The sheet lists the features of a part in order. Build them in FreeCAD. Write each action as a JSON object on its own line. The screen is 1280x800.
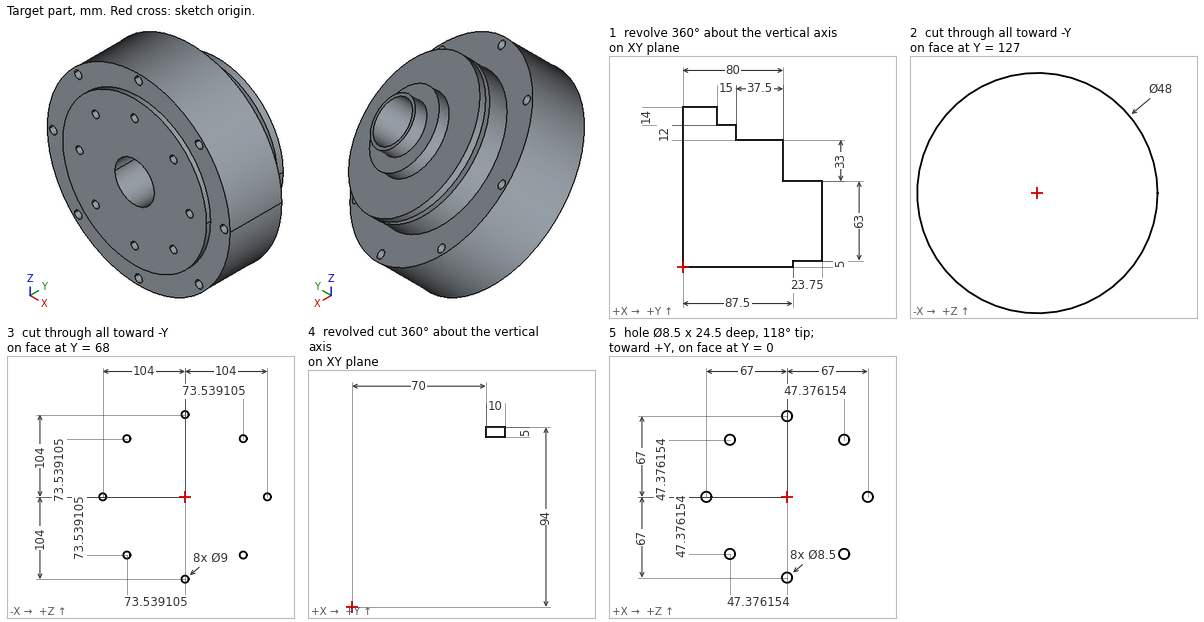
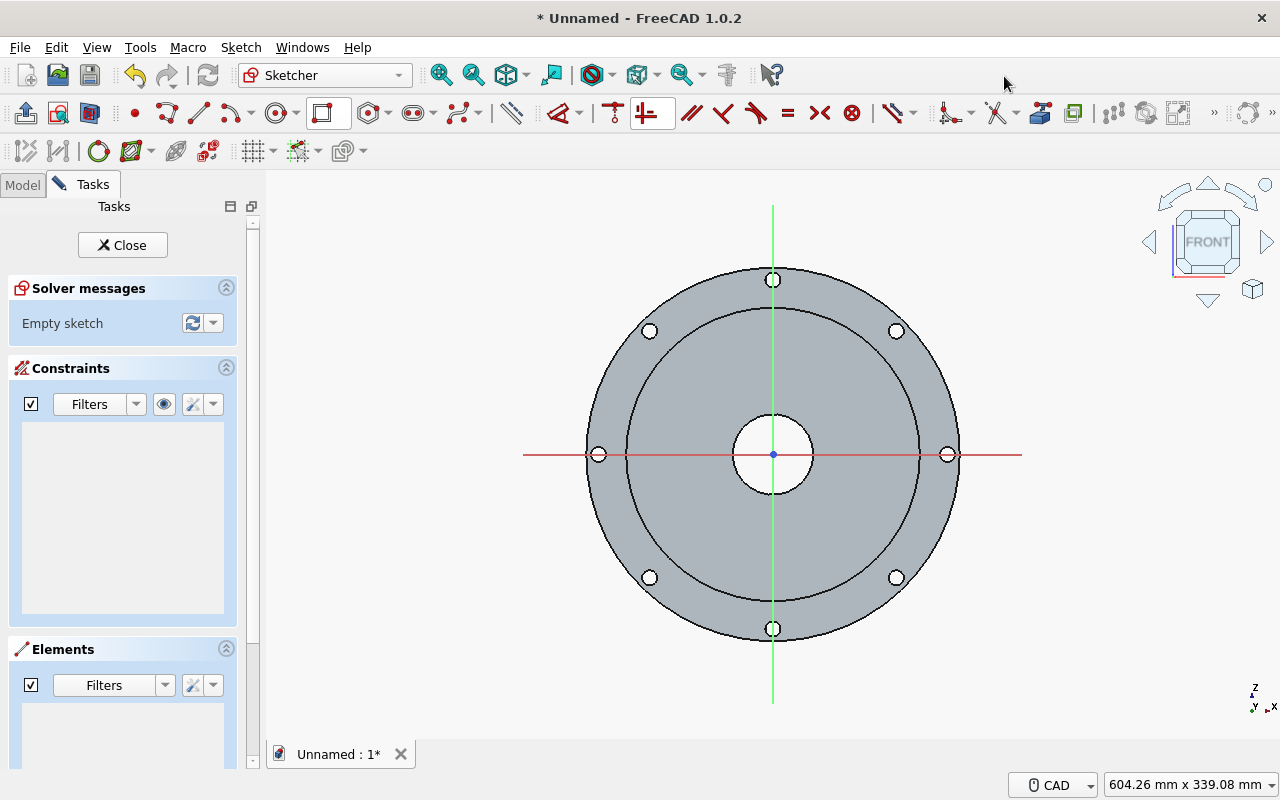
{"action": "scroll", "coordinate": [912, 455], "scroll_direction": "up", "scroll_amount": 2}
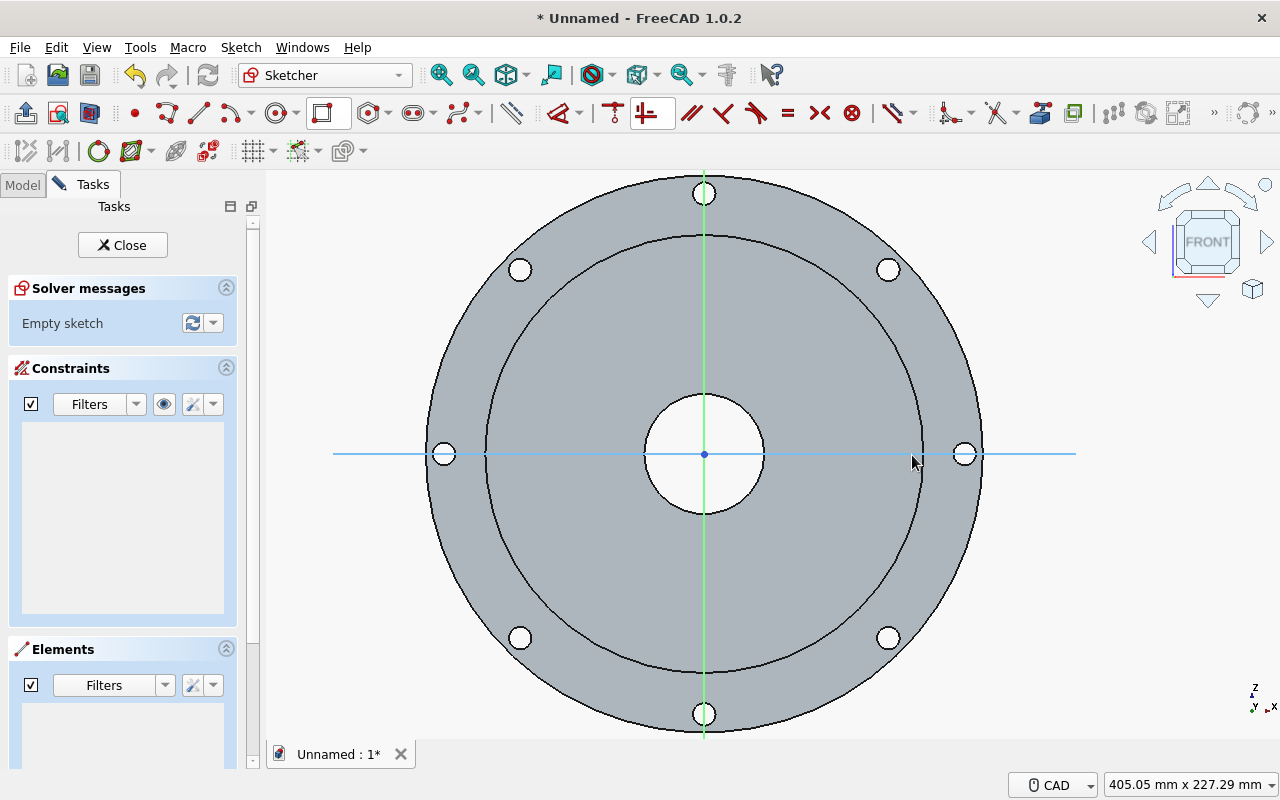
{"action": "left_click", "coordinate": [276, 114]}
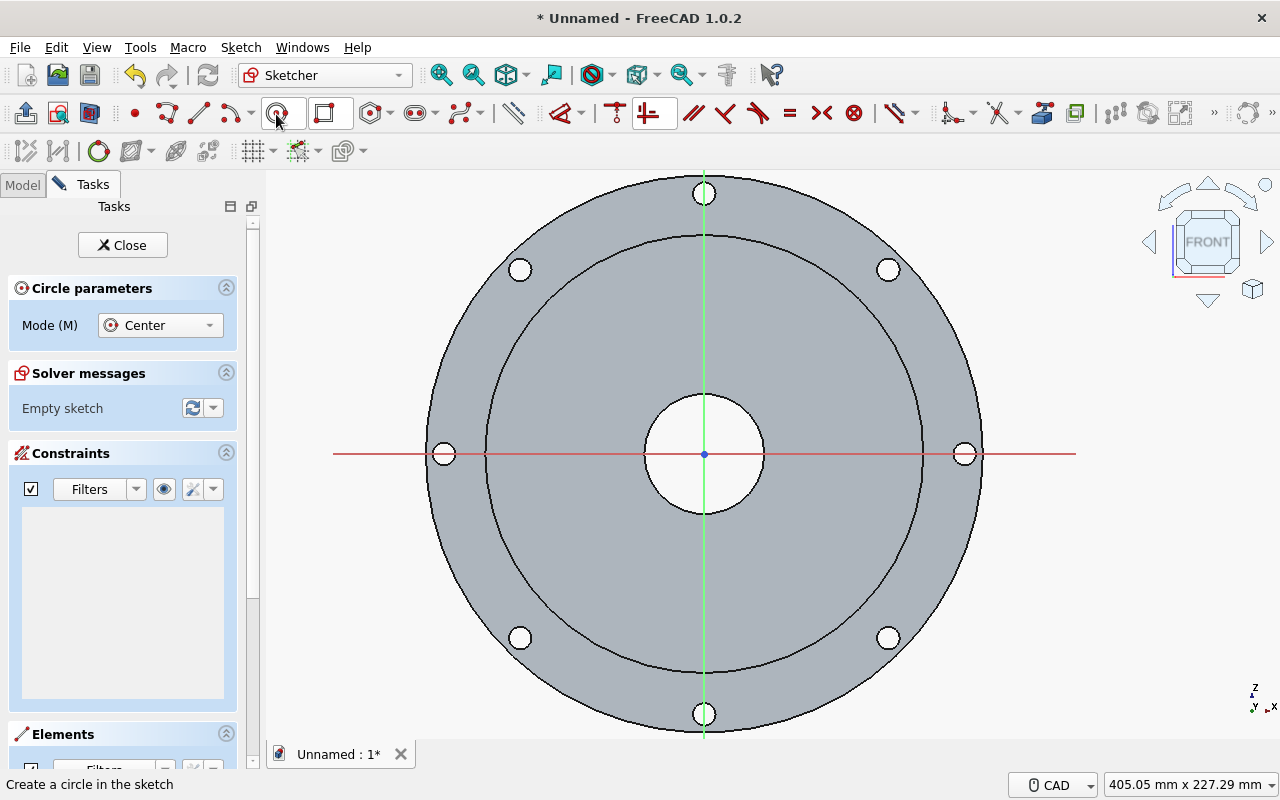
{"action": "scroll", "coordinate": [704, 622], "scroll_direction": "up", "scroll_amount": 4}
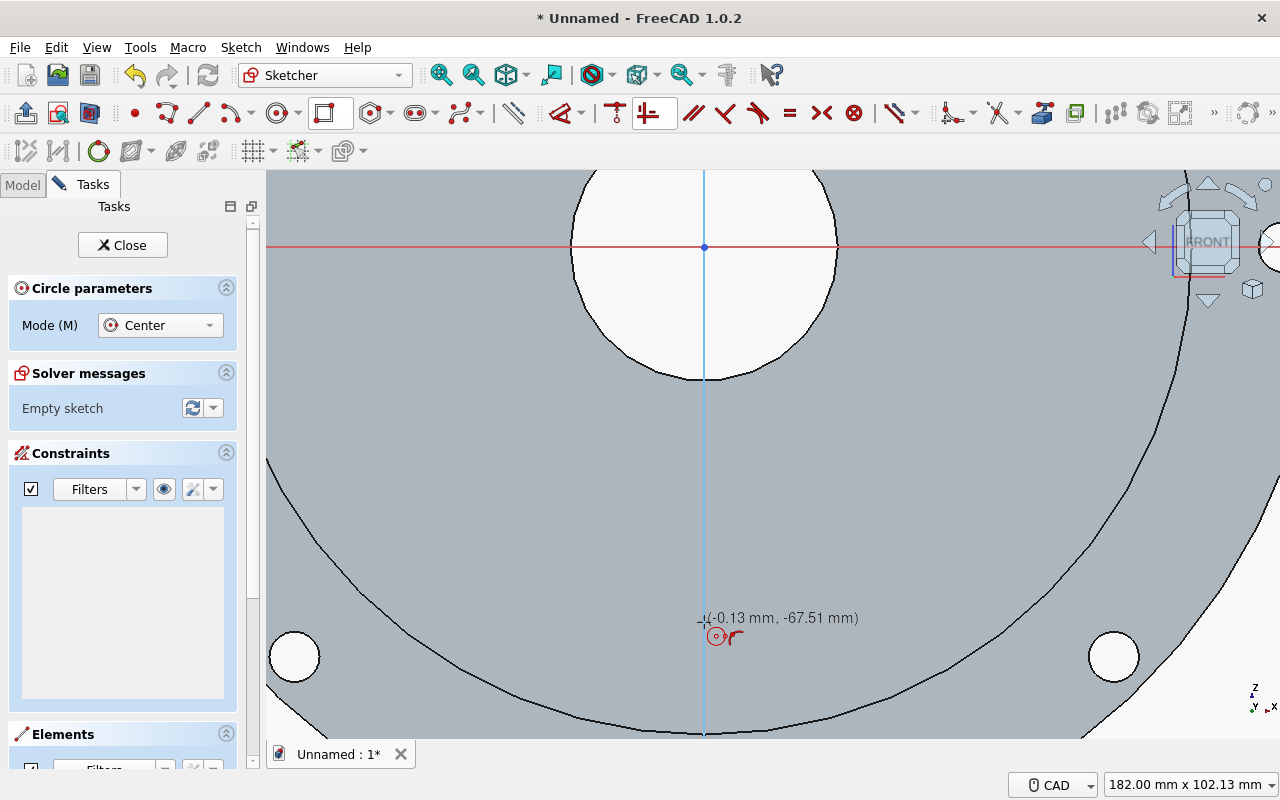
{"action": "left_click", "coordinate": [704, 620]}
{"action": "left_click", "coordinate": [721, 604]}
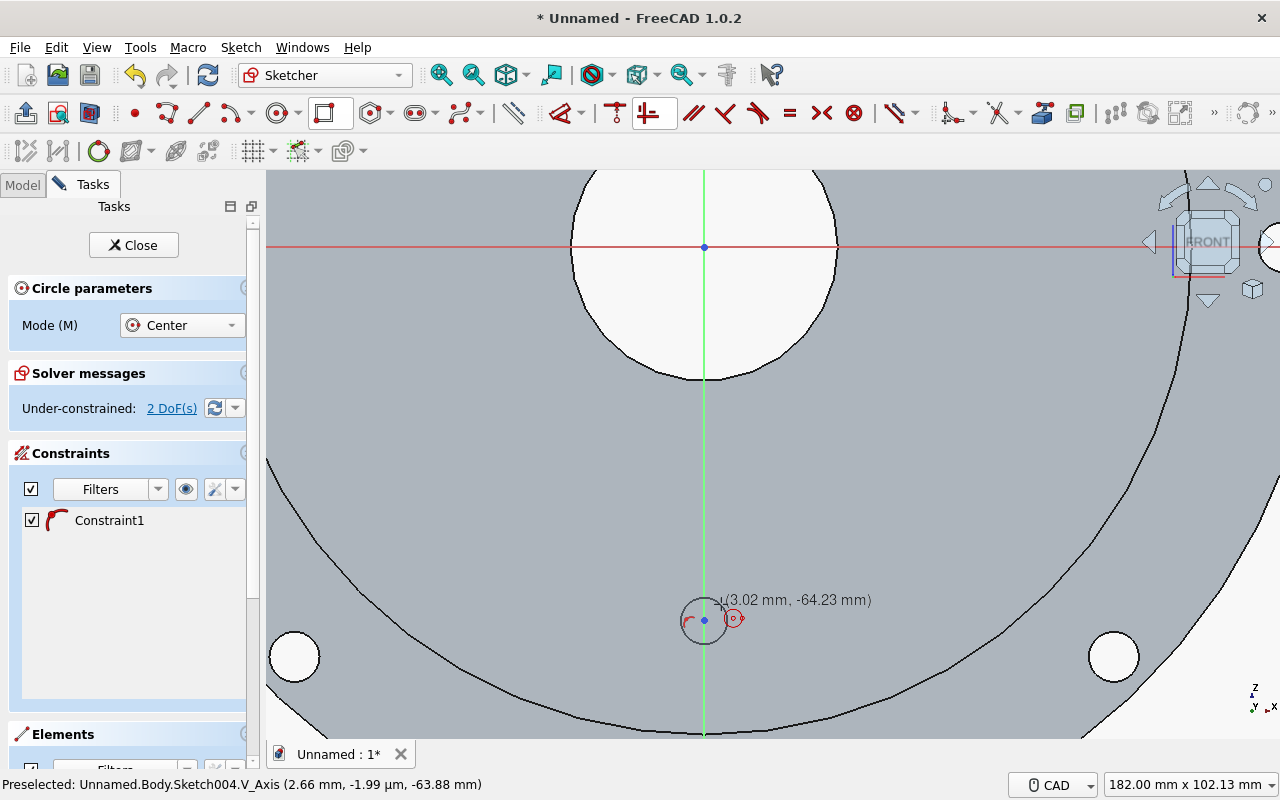
{"action": "left_click", "coordinate": [440, 511]}
{"action": "left_click", "coordinate": [457, 494]}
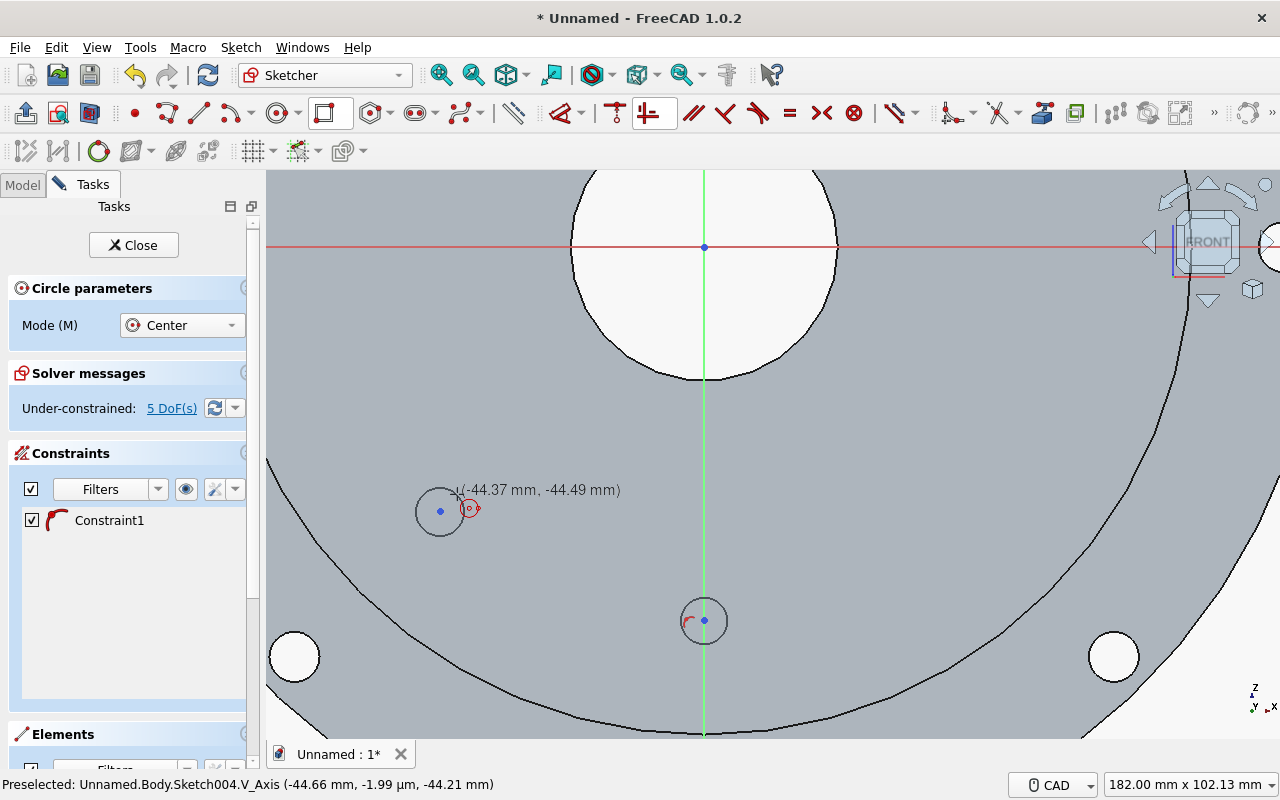
{"action": "left_click", "coordinate": [331, 247]}
{"action": "left_click", "coordinate": [348, 230]}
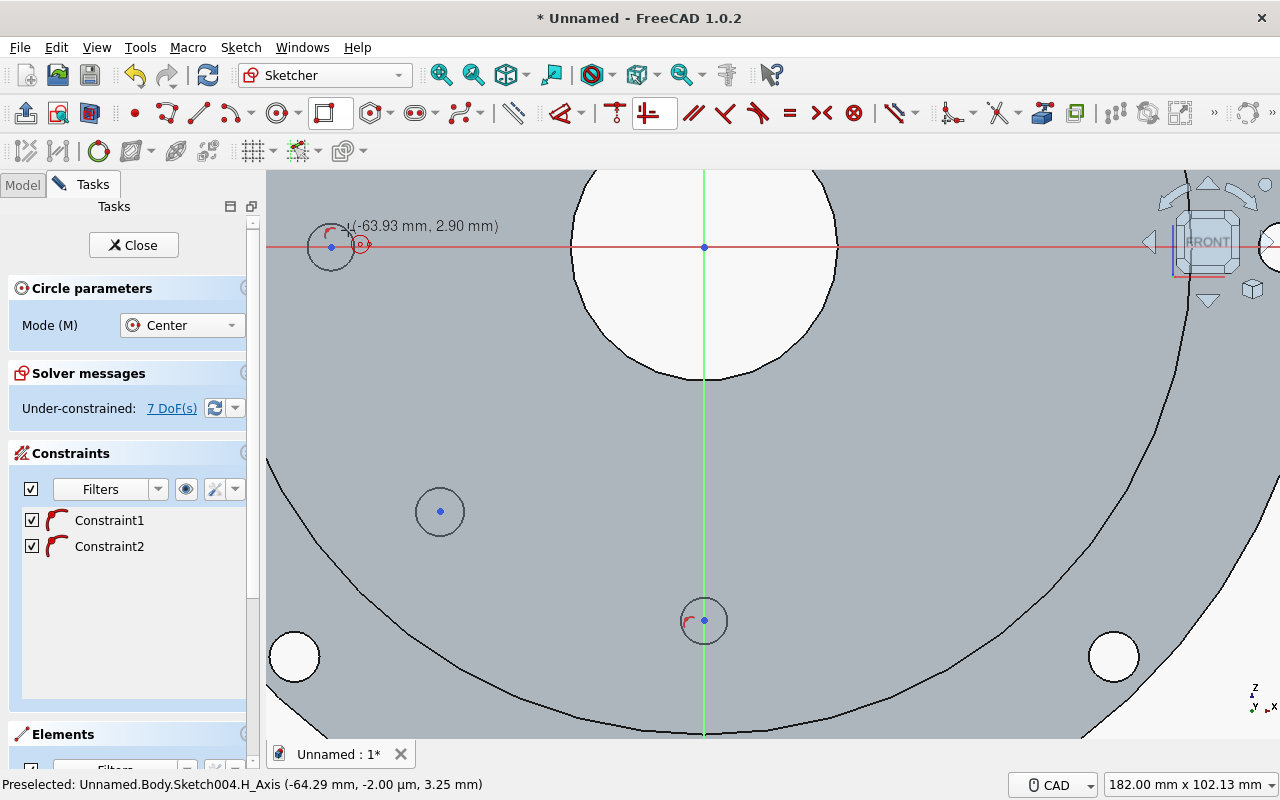
{"action": "scroll", "coordinate": [705, 624], "scroll_direction": "down", "scroll_amount": 4}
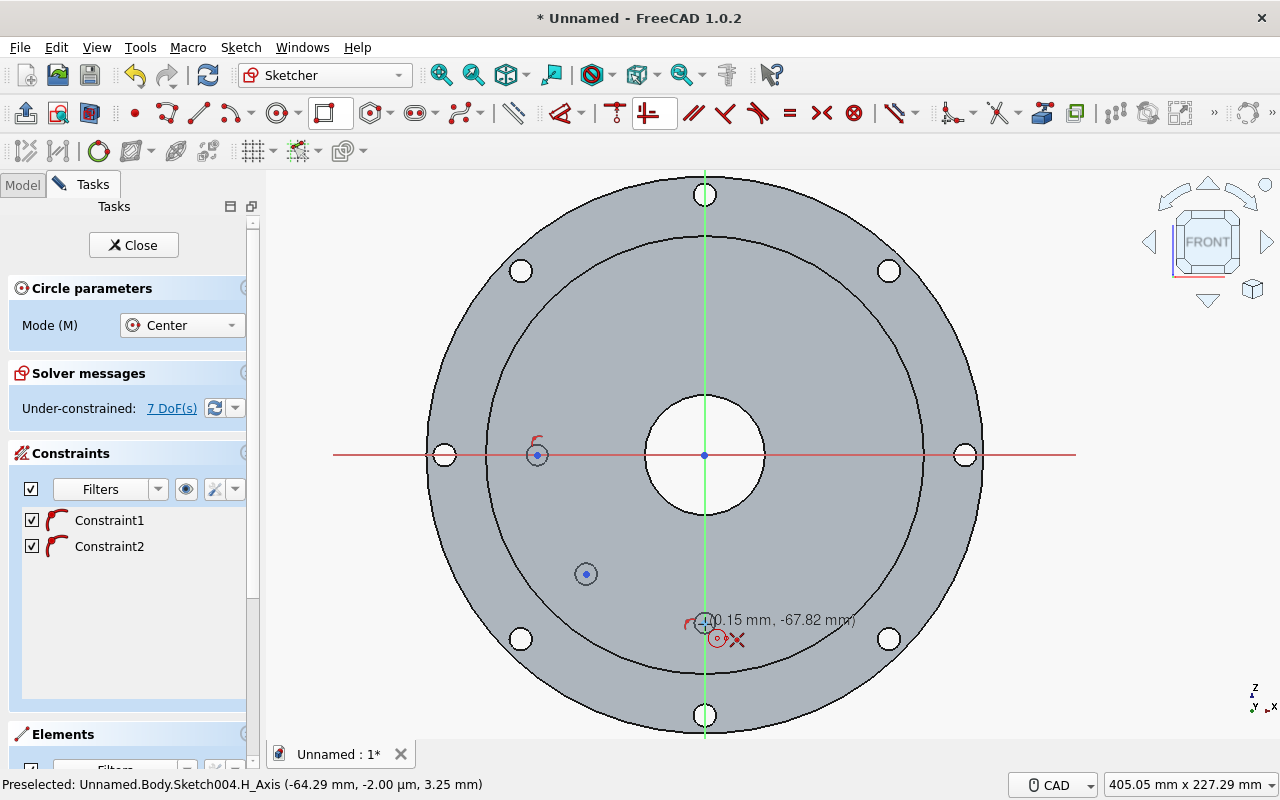
{"action": "scroll", "coordinate": [586, 337], "scroll_direction": "up", "scroll_amount": 4}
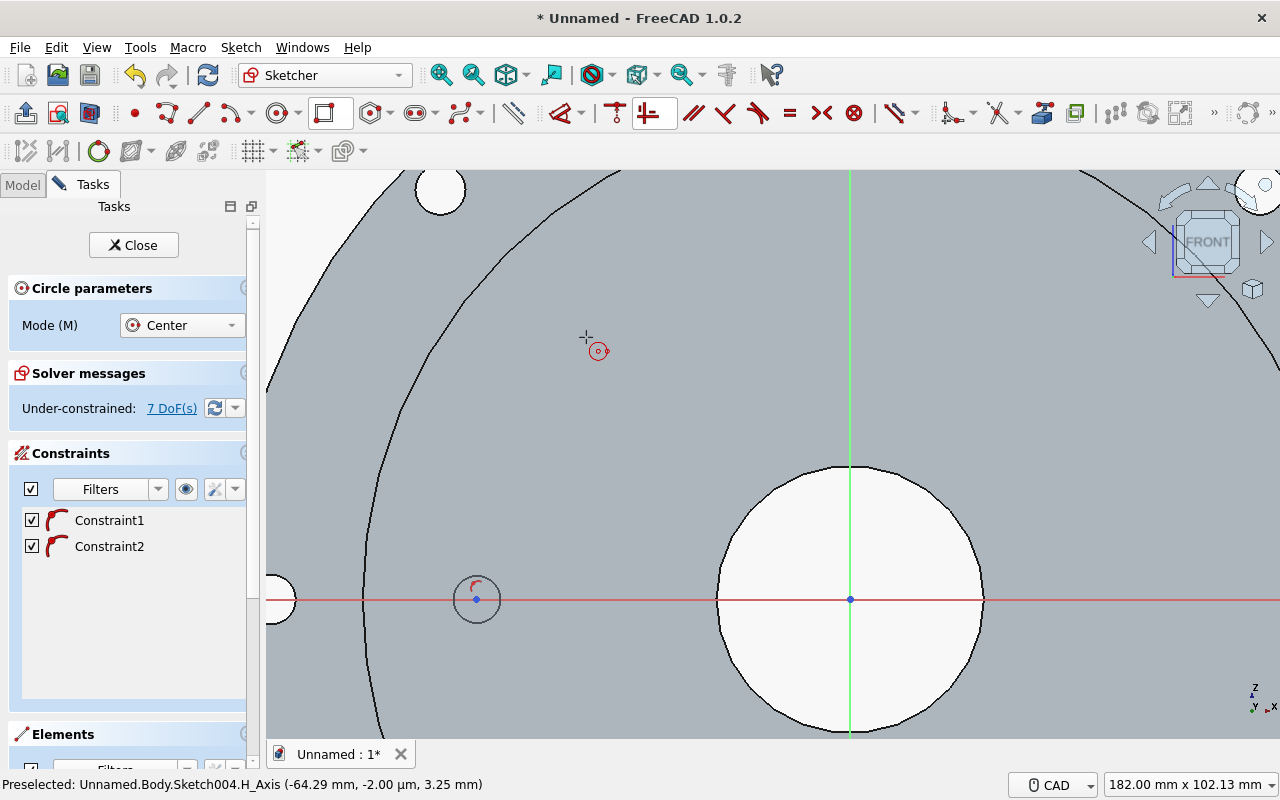
{"action": "left_click", "coordinate": [586, 336]}
{"action": "left_click", "coordinate": [603, 319]}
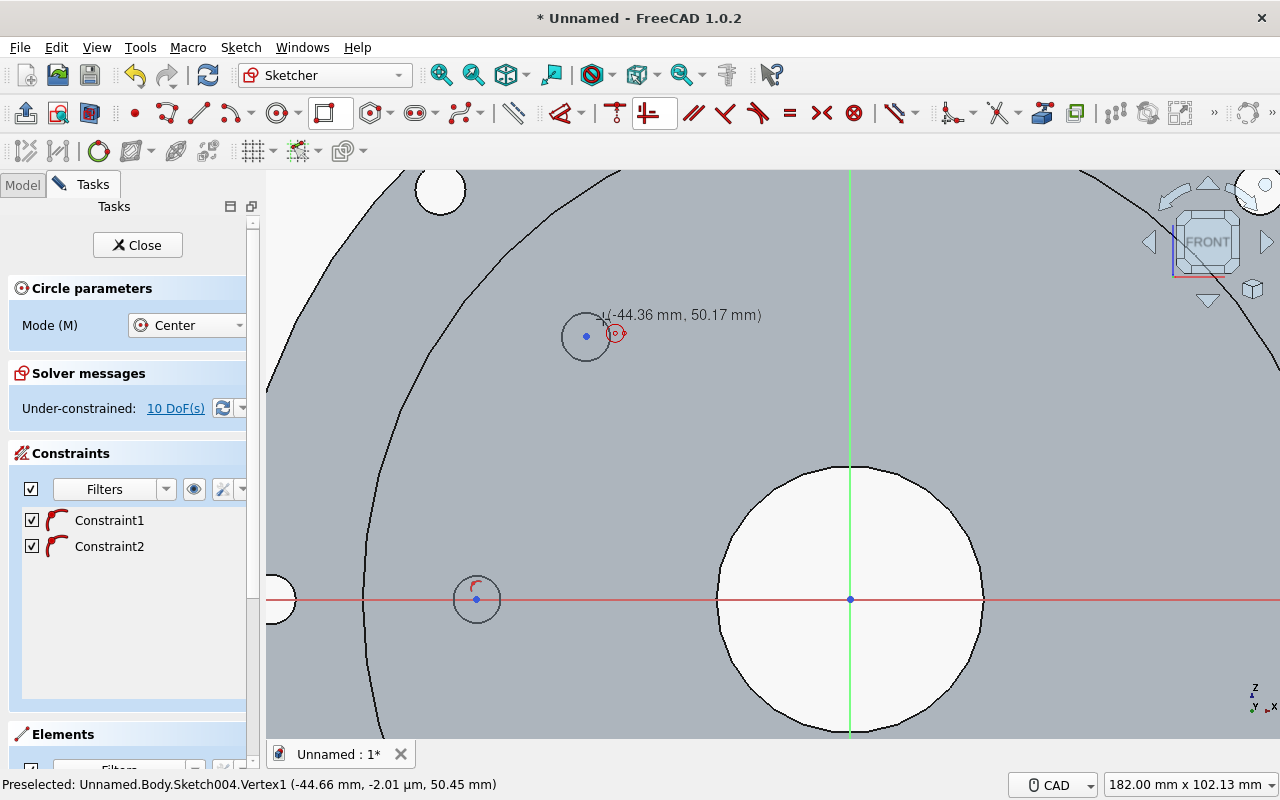
{"action": "left_click", "coordinate": [850, 226]}
{"action": "left_click", "coordinate": [867, 209]}